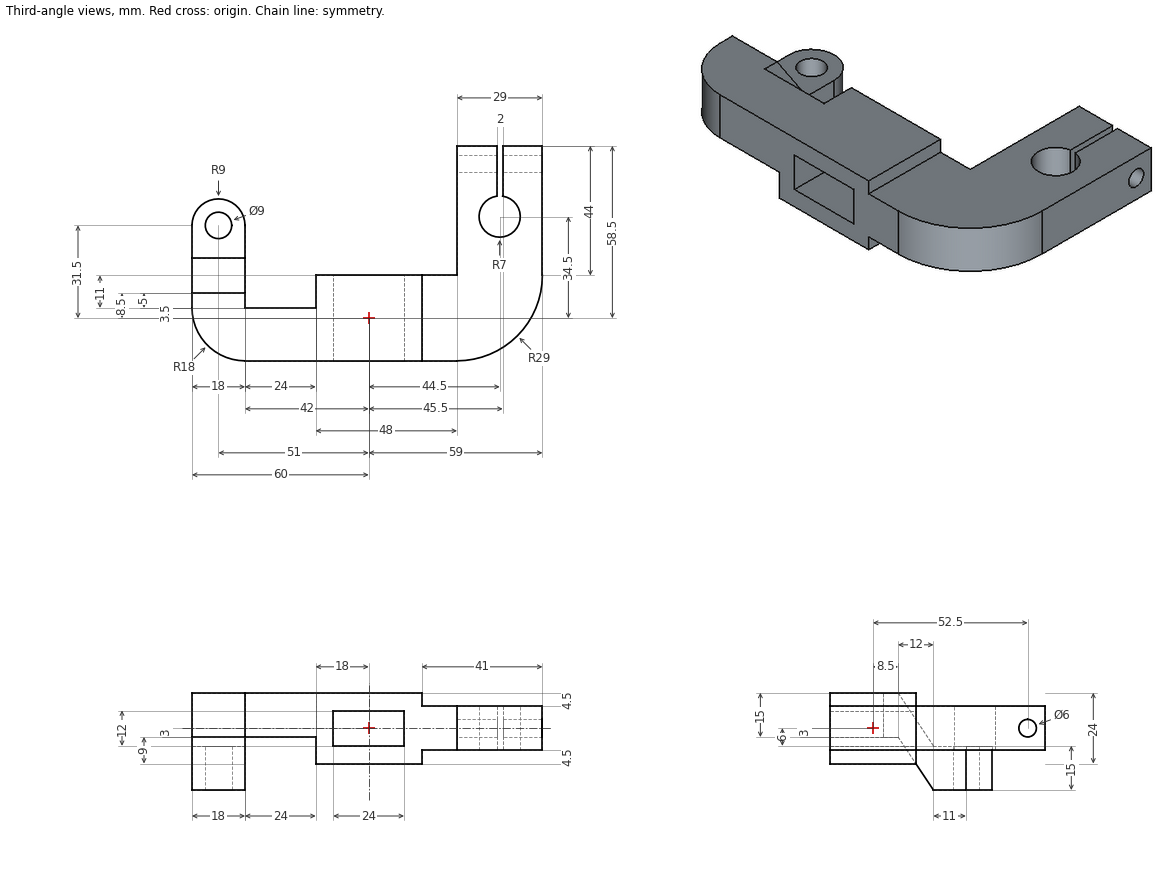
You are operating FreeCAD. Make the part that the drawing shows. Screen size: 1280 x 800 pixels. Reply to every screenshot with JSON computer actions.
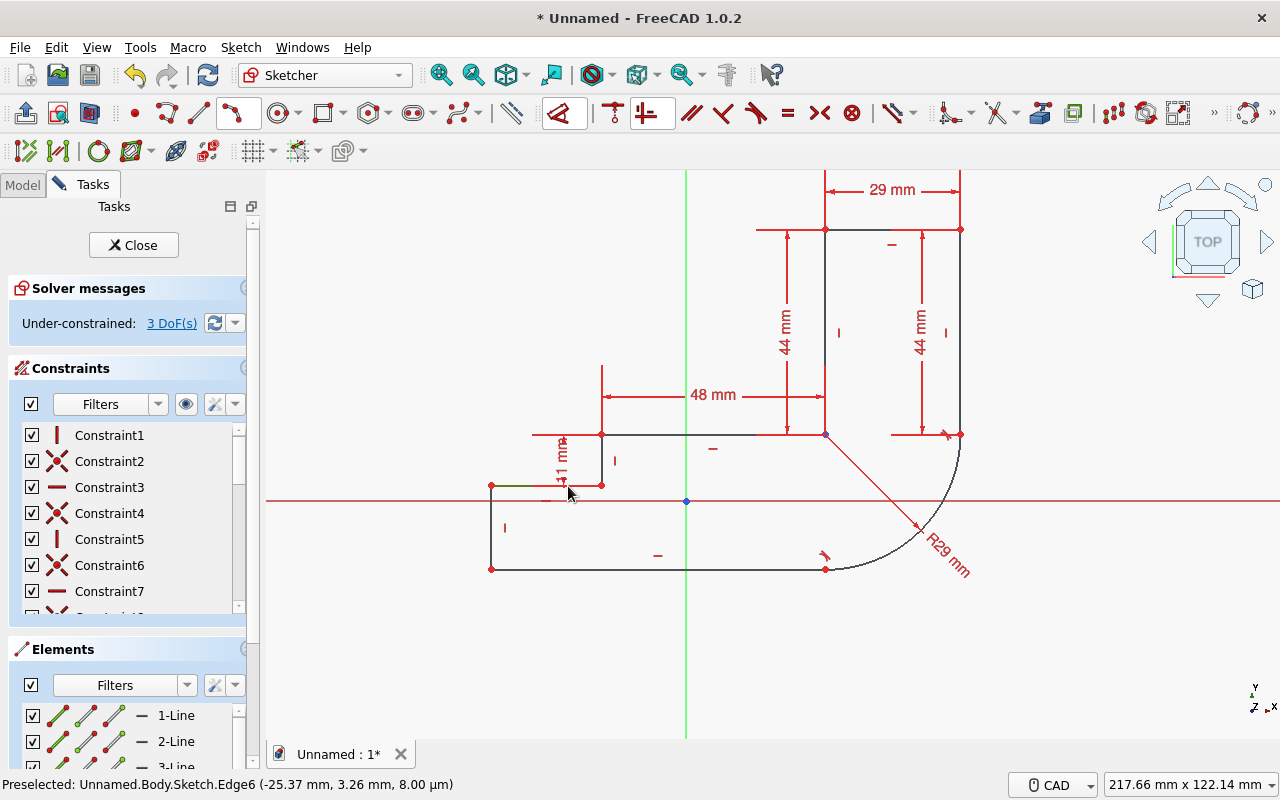
{"action": "left_click", "coordinate": [582, 114]}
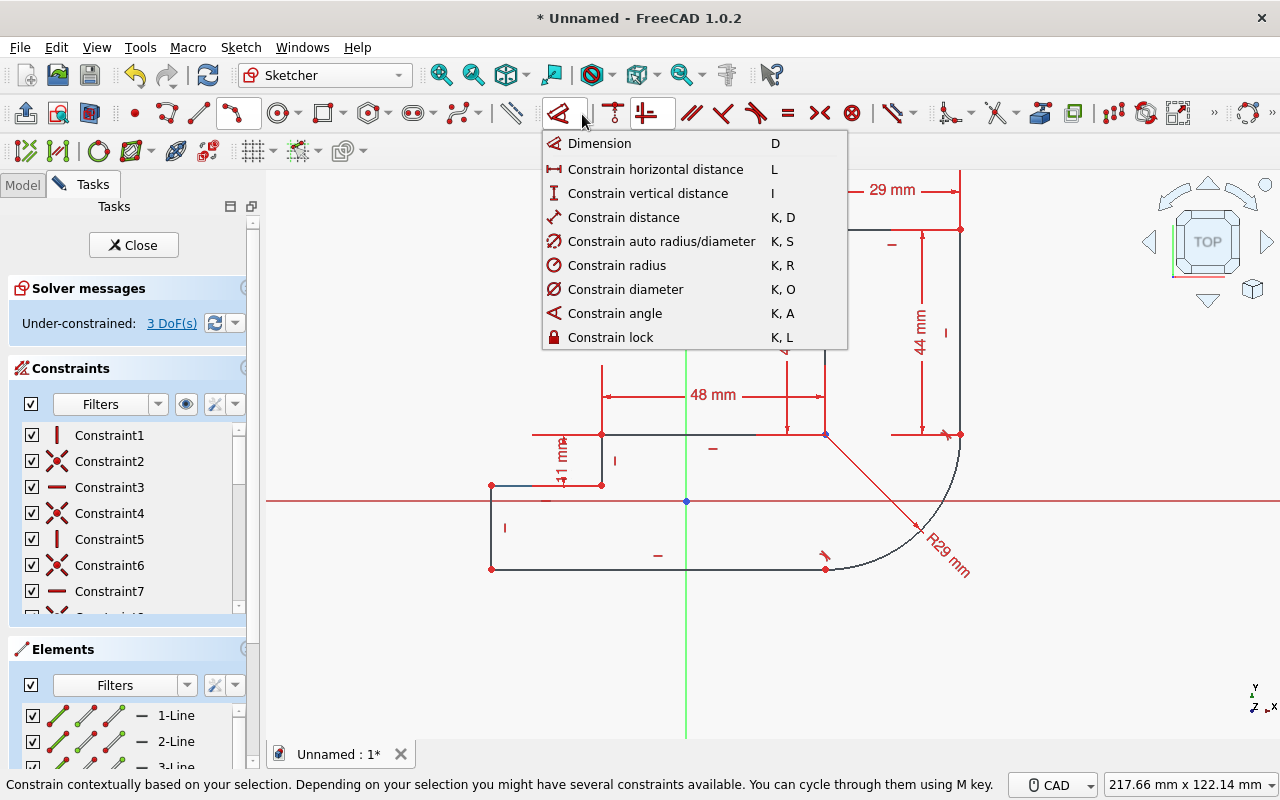
{"action": "left_click", "coordinate": [695, 169]}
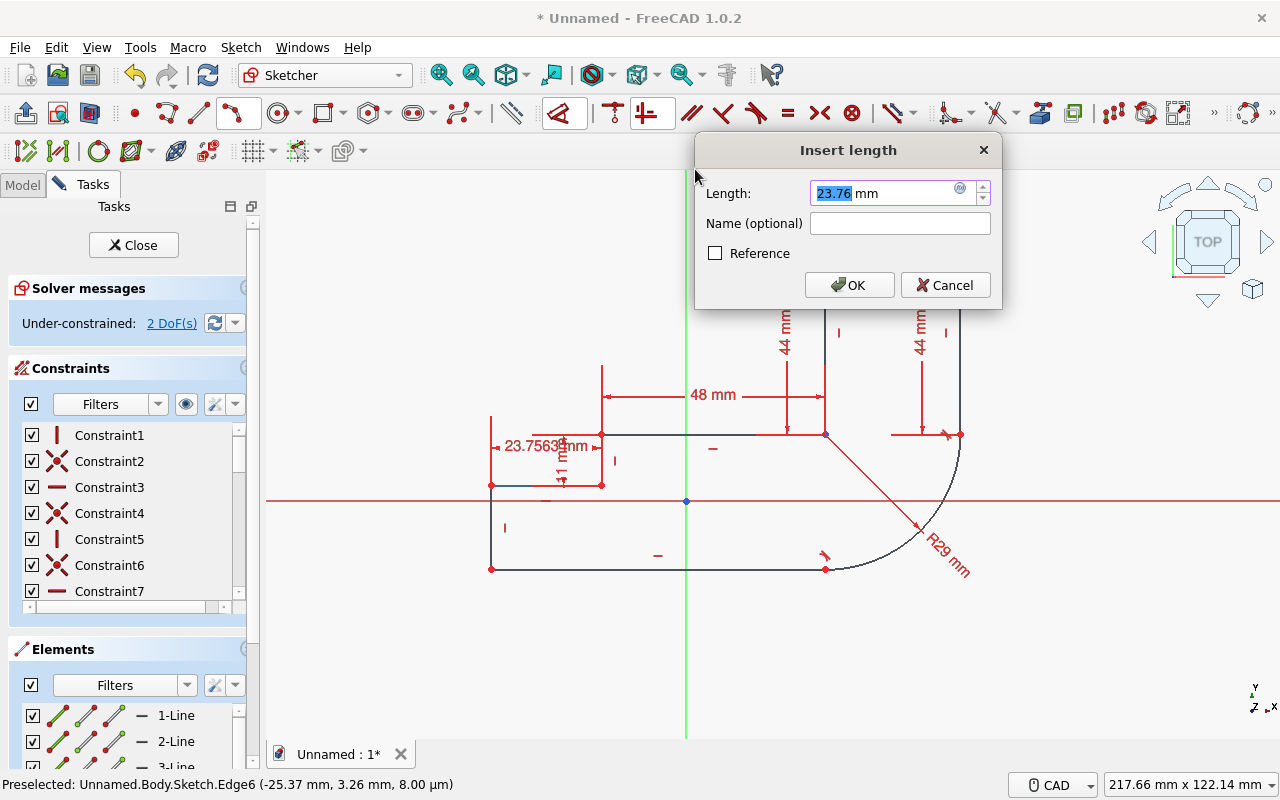
{"action": "type", "text": "24"}
{"action": "key", "text": "Return"}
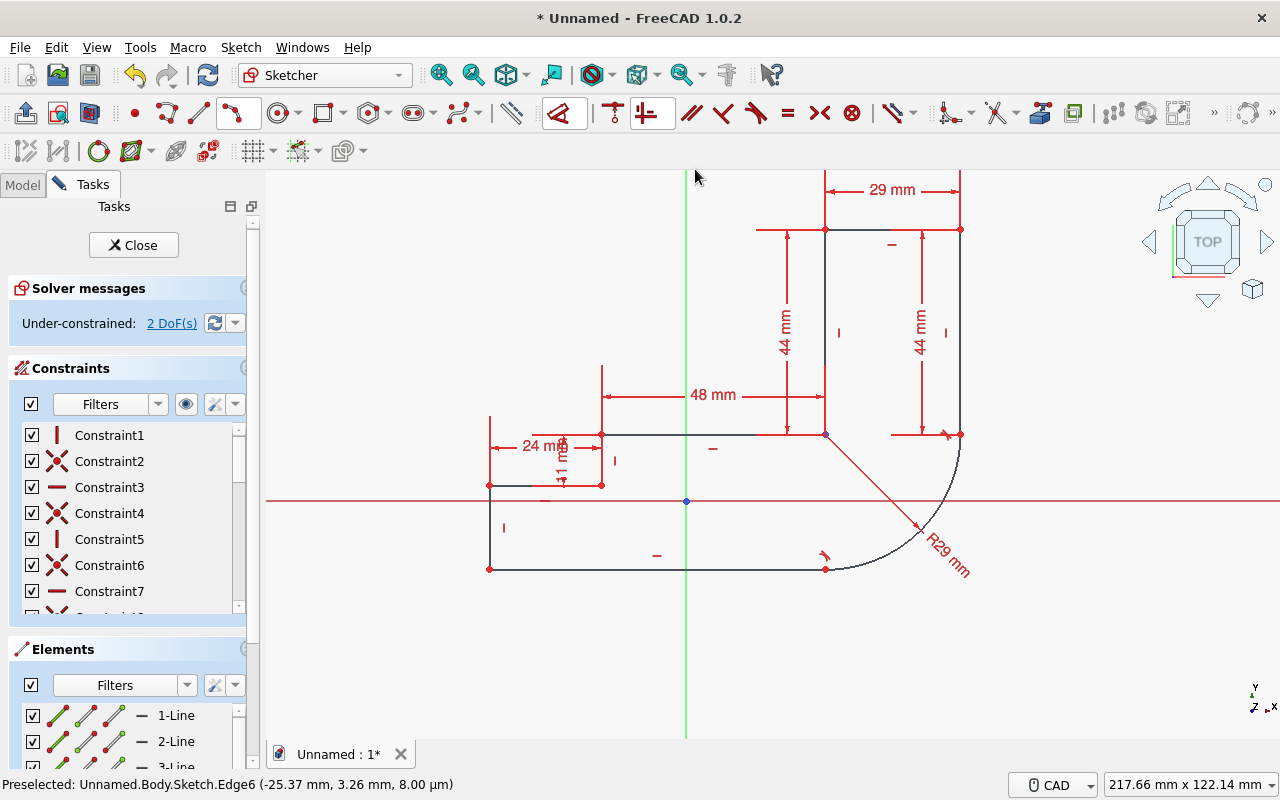
{"action": "left_click", "coordinate": [960, 435]}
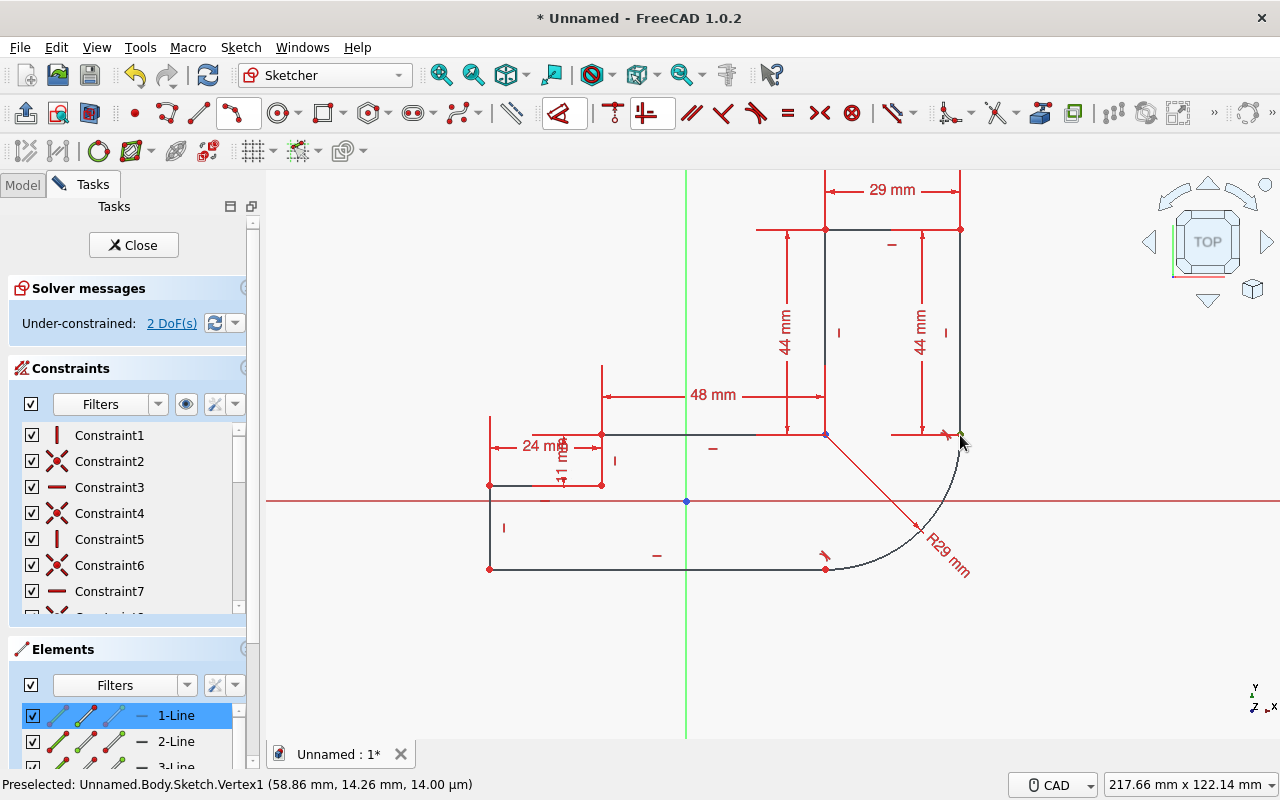
{"action": "key", "text": "l"}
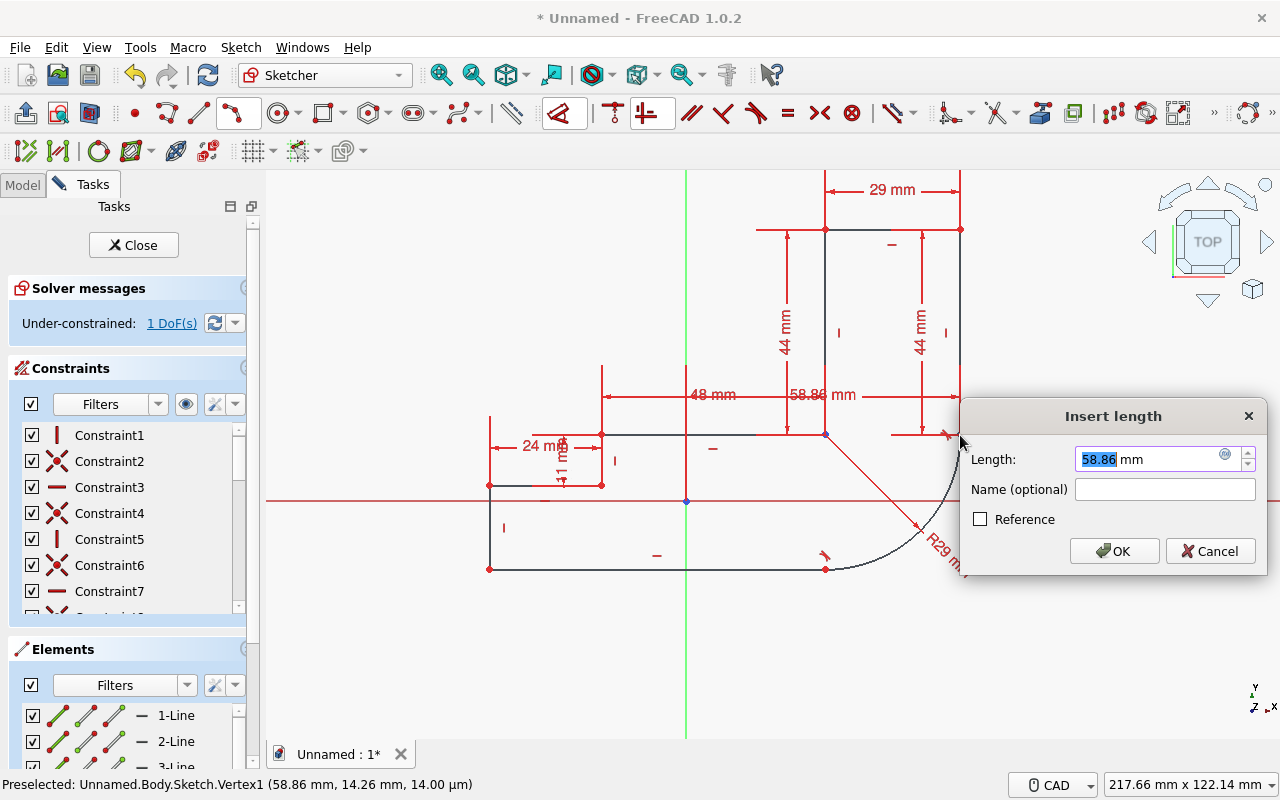
{"action": "type", "text": "59"}
{"action": "key", "text": "Return"}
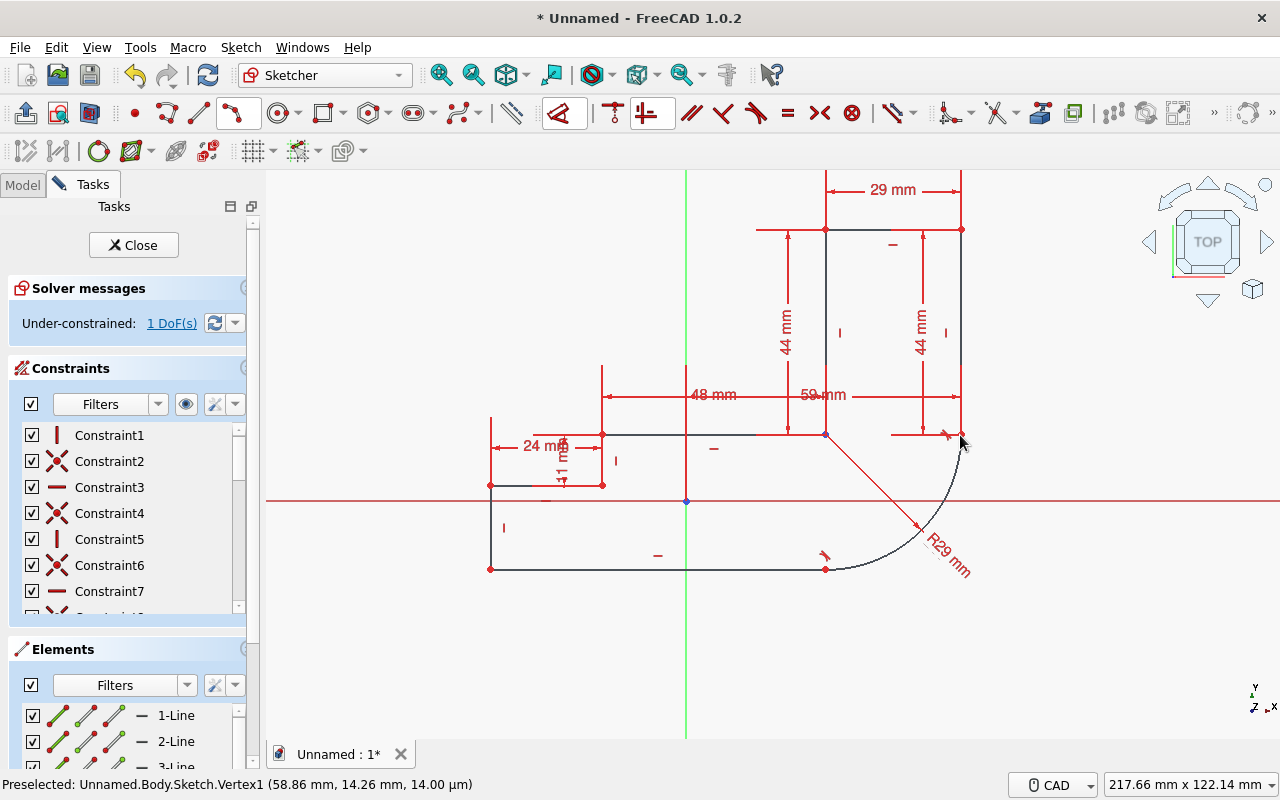
{"action": "scroll", "coordinate": [602, 486], "scroll_direction": "up", "scroll_amount": 5}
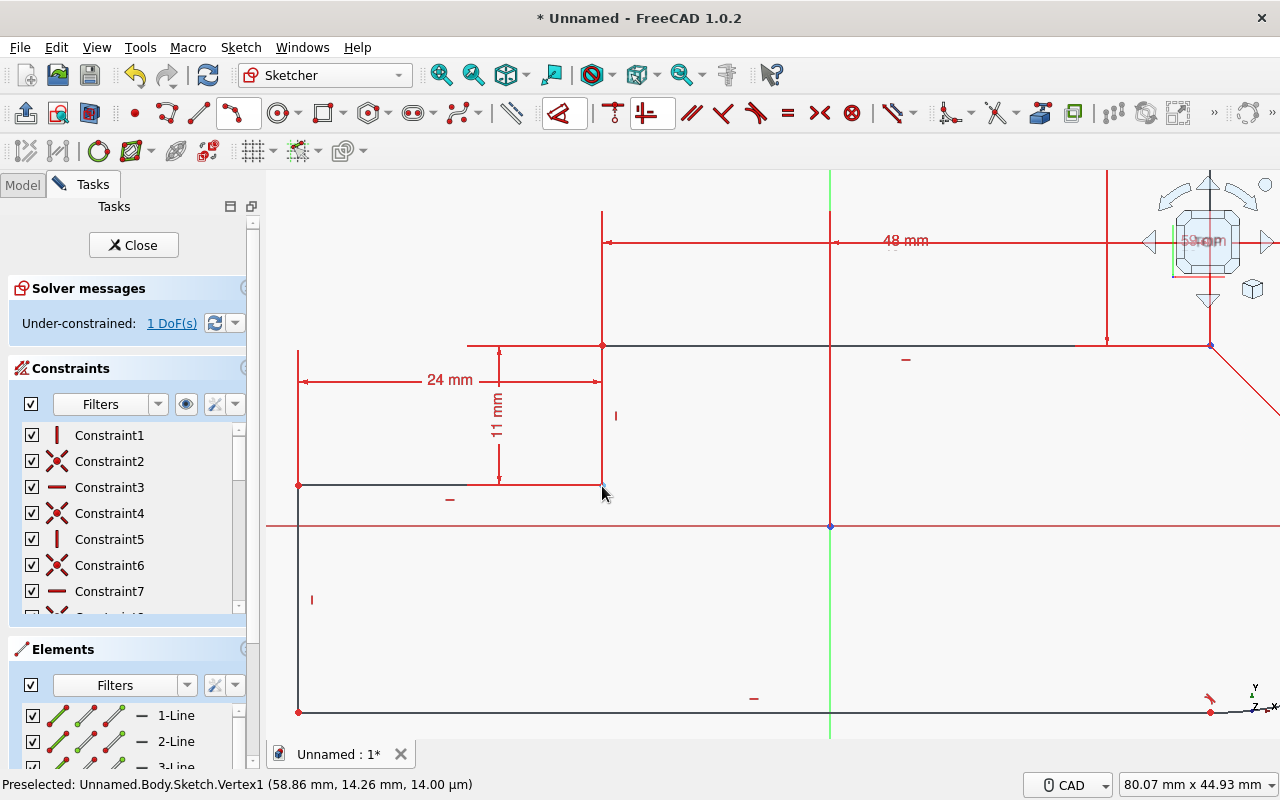
{"action": "left_click", "coordinate": [602, 485]}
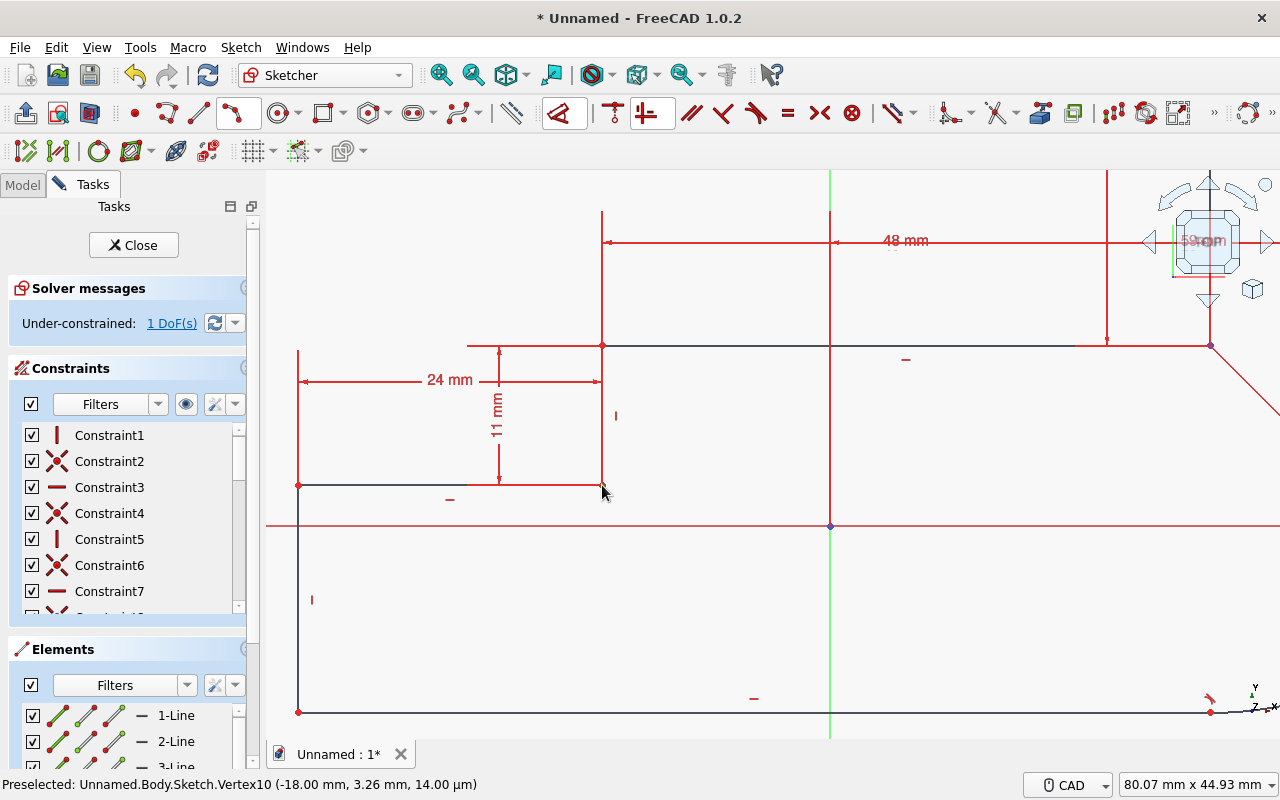
{"action": "key", "text": "i"}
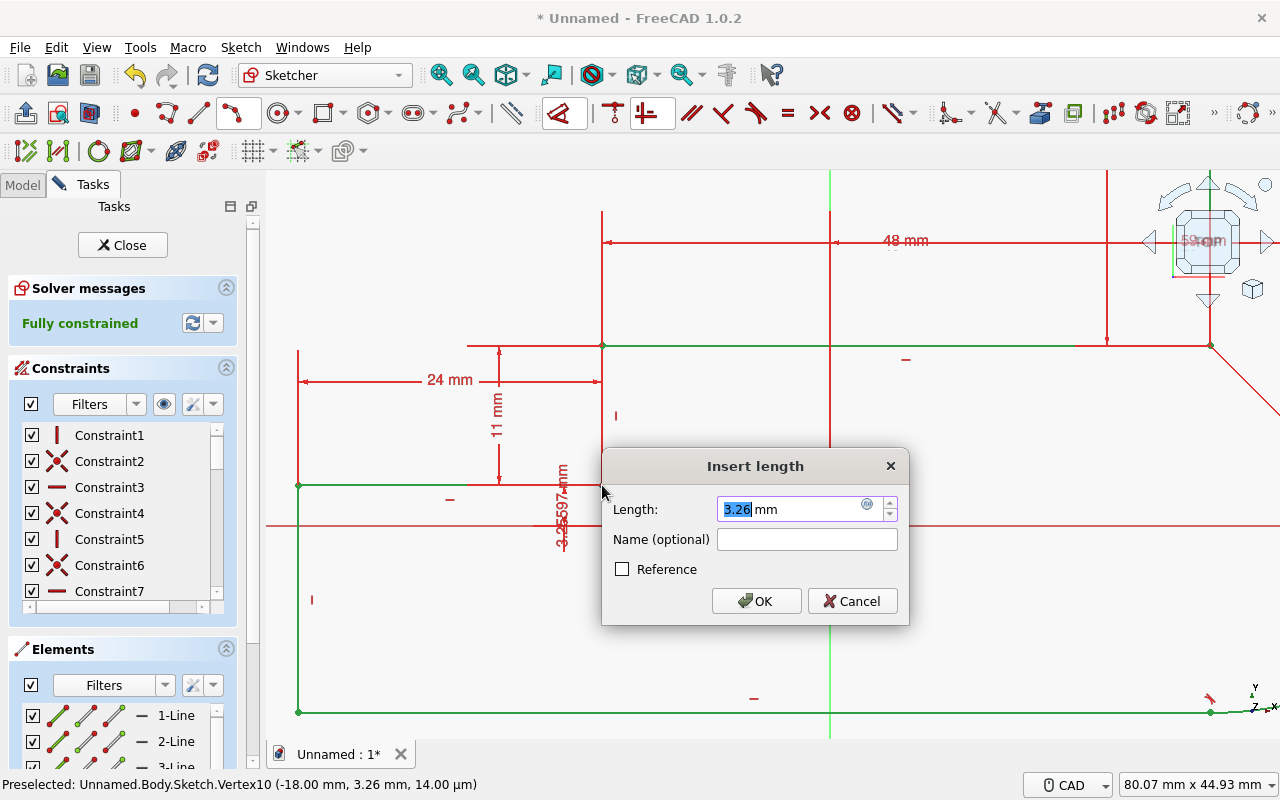
{"action": "type", "text": "3.5"}
{"action": "key", "text": "Return"}